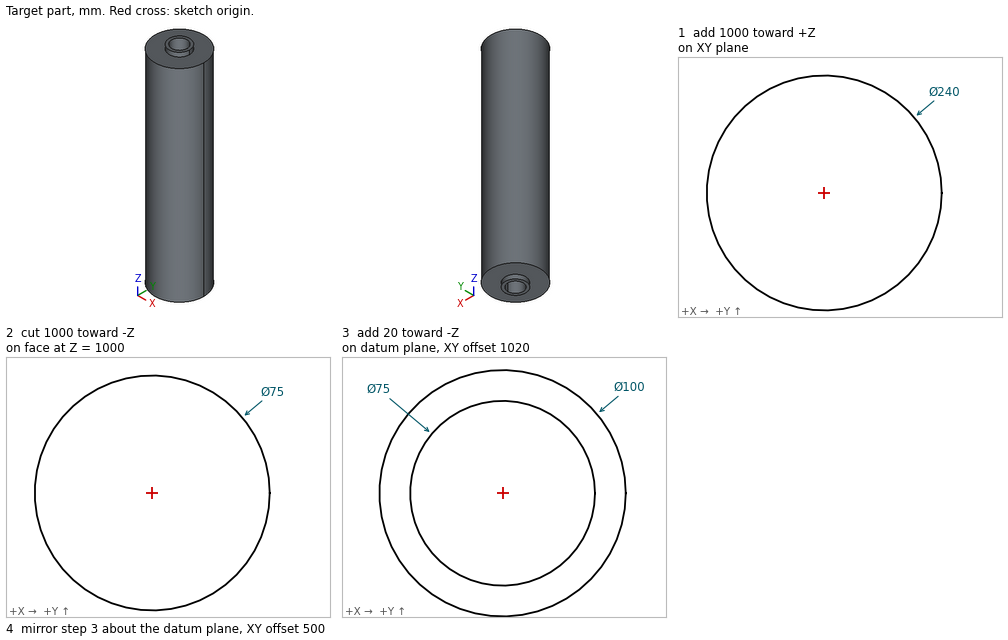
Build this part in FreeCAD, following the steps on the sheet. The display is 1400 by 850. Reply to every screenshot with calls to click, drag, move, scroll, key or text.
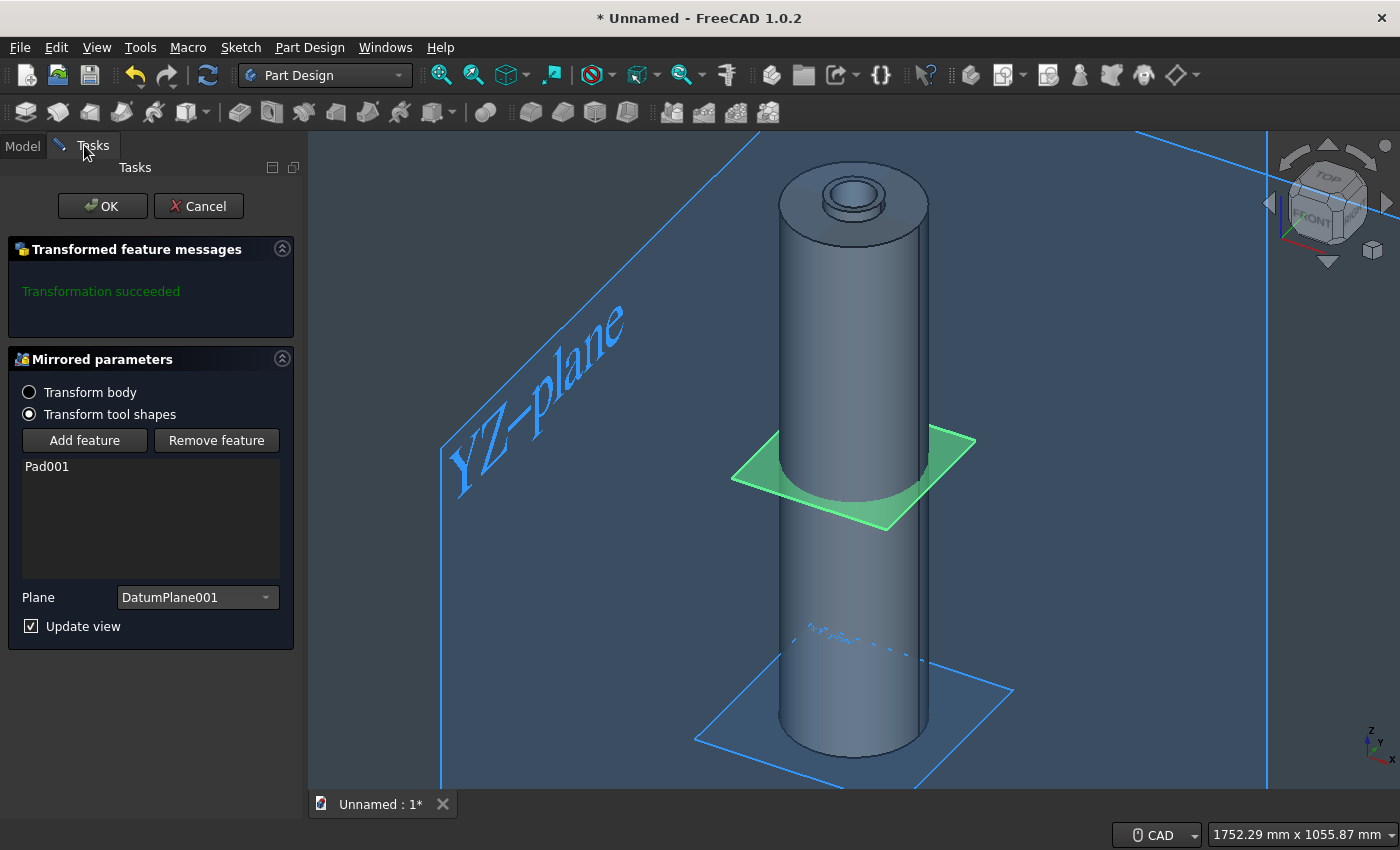
click(103, 206)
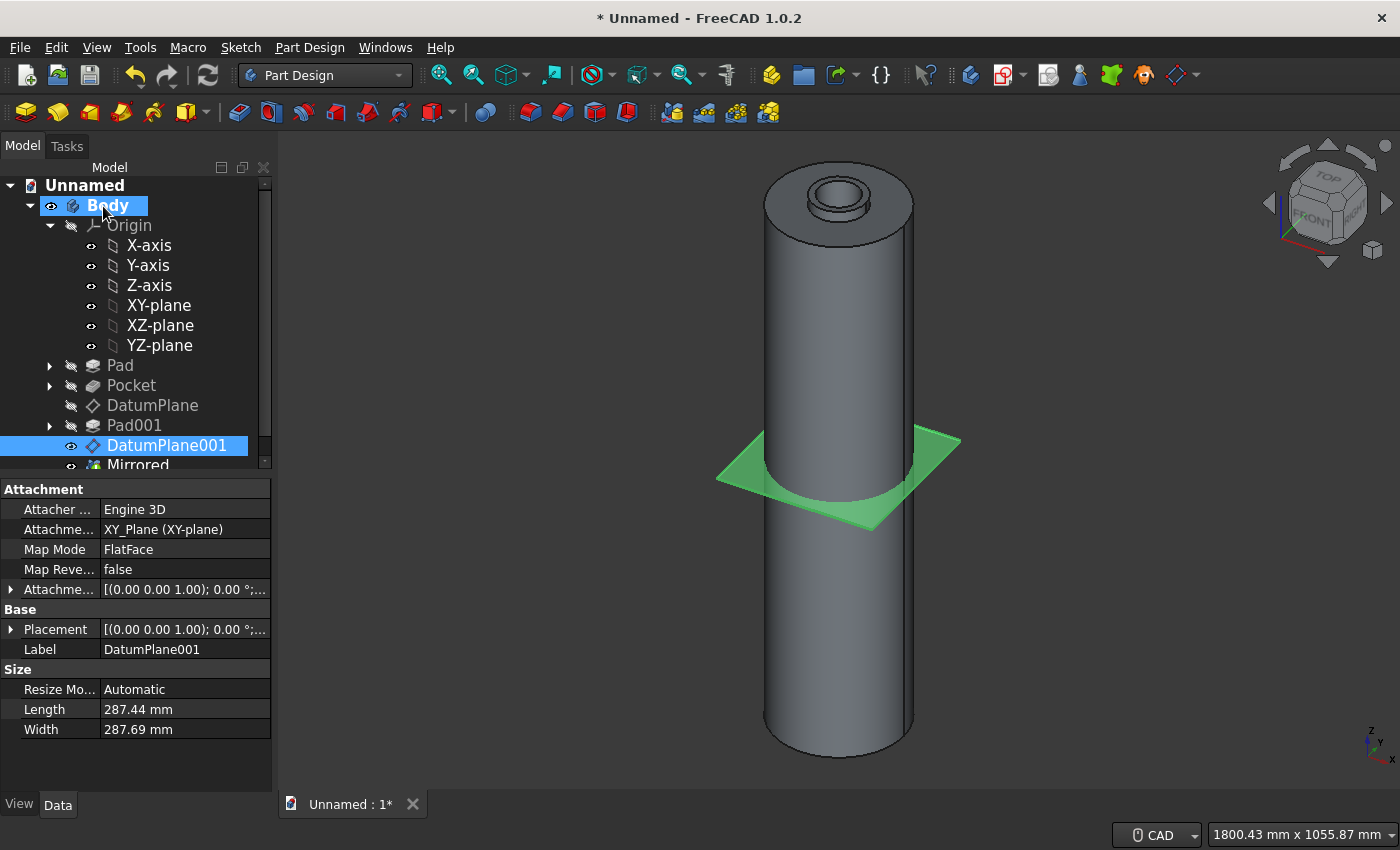
click(116, 446)
key(space)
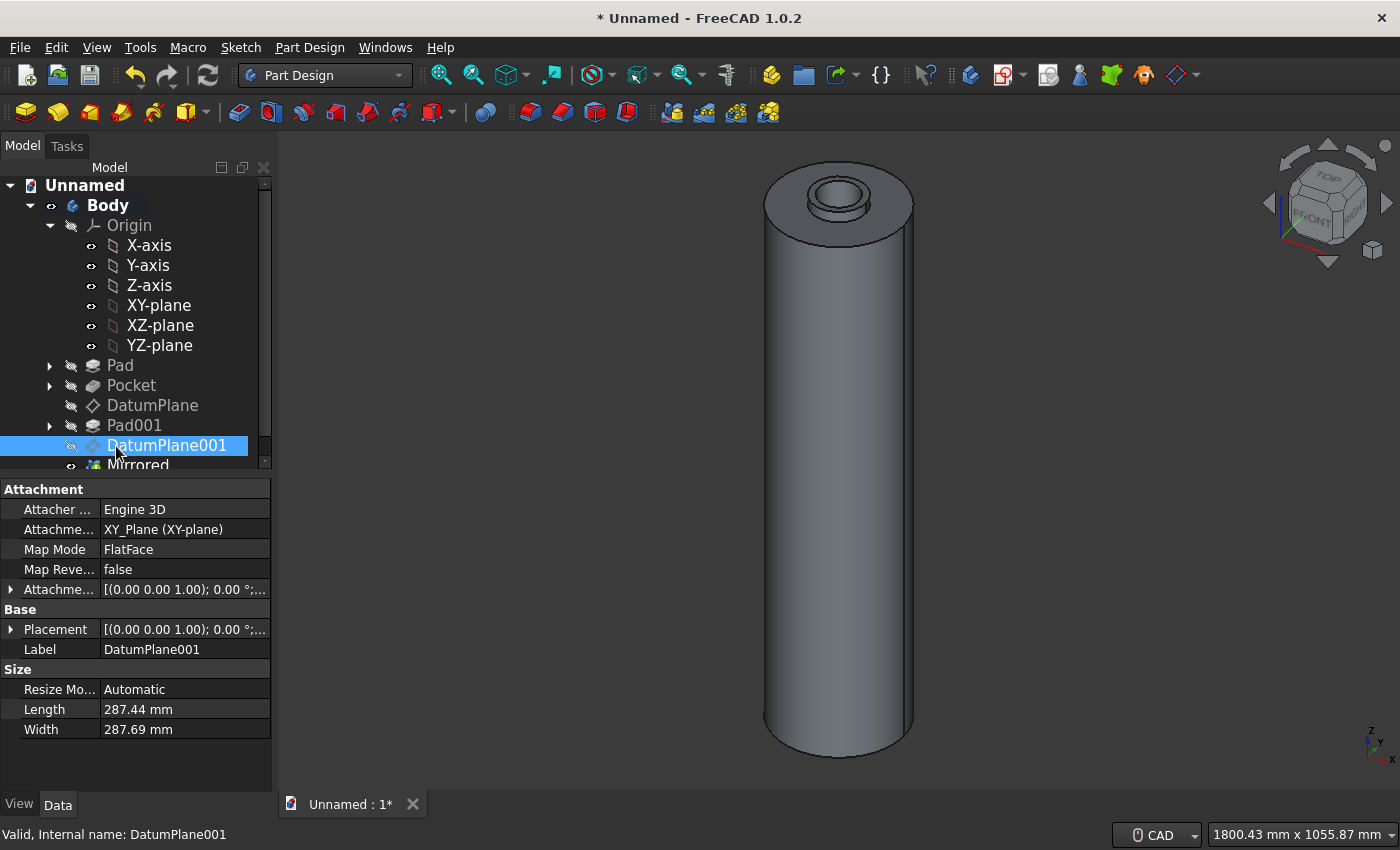
key(0)